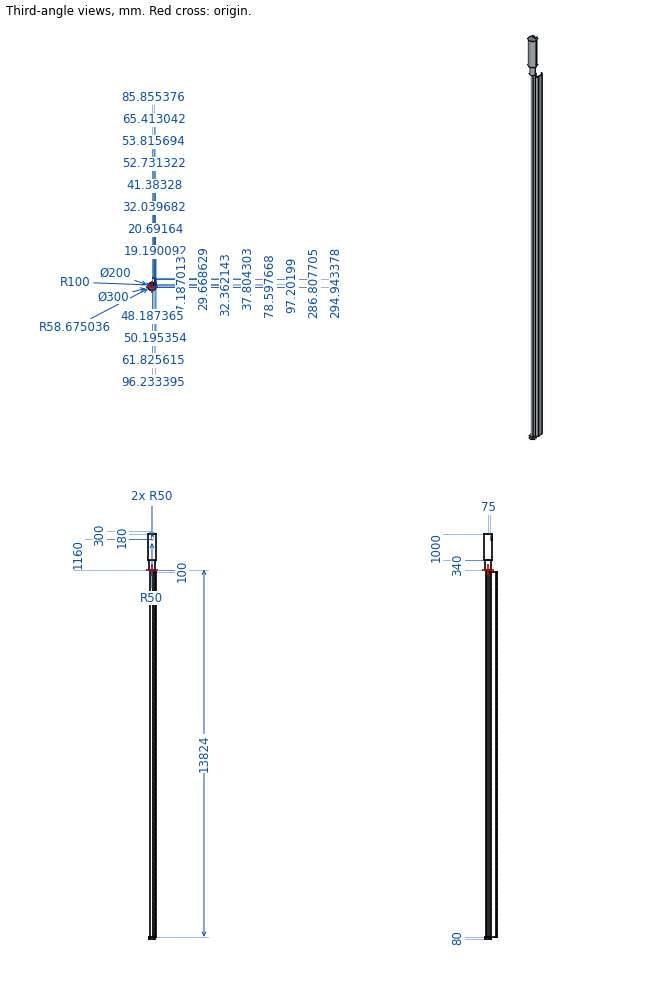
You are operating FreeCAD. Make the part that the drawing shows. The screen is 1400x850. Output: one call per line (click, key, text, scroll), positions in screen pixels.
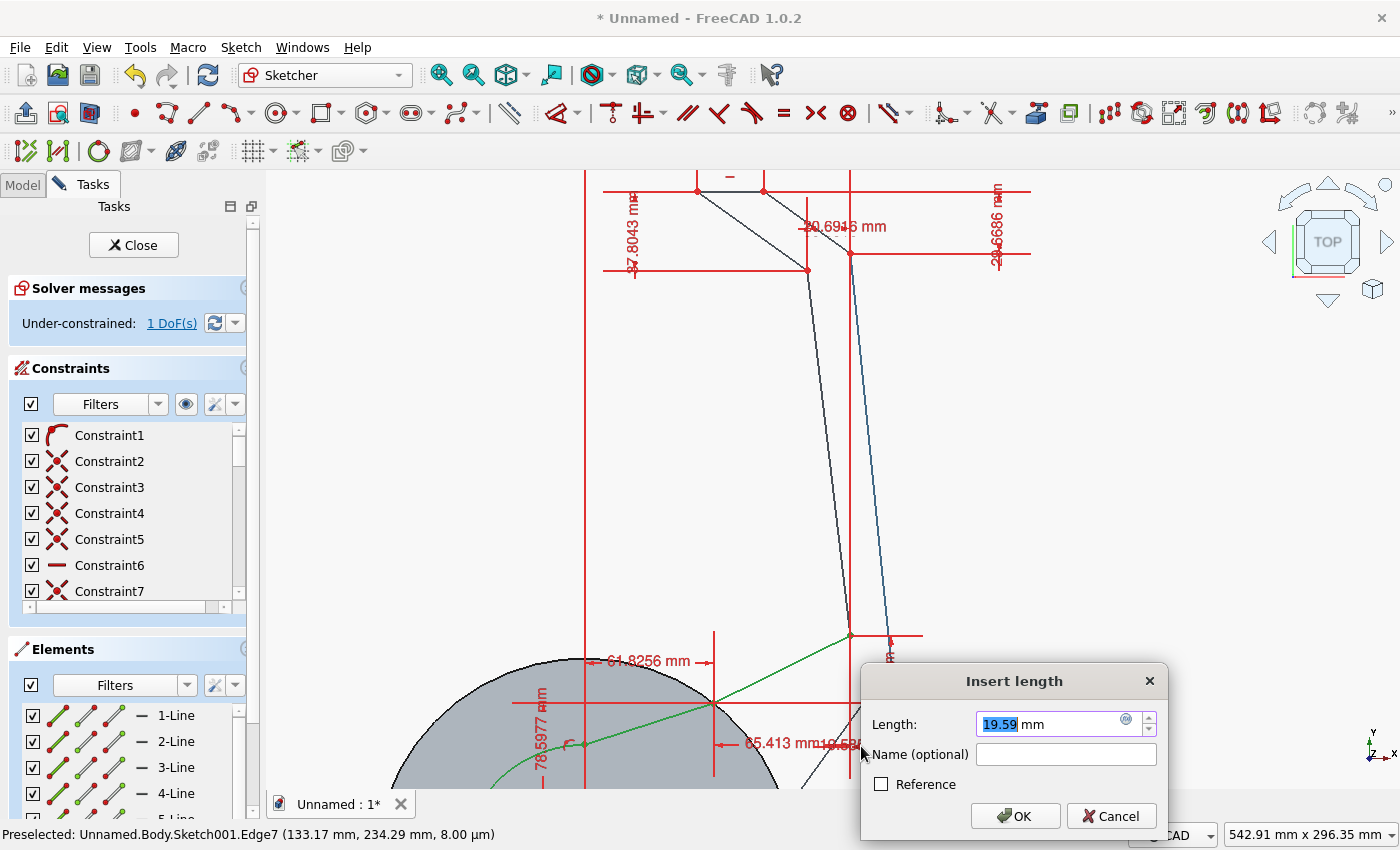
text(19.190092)
key(Return)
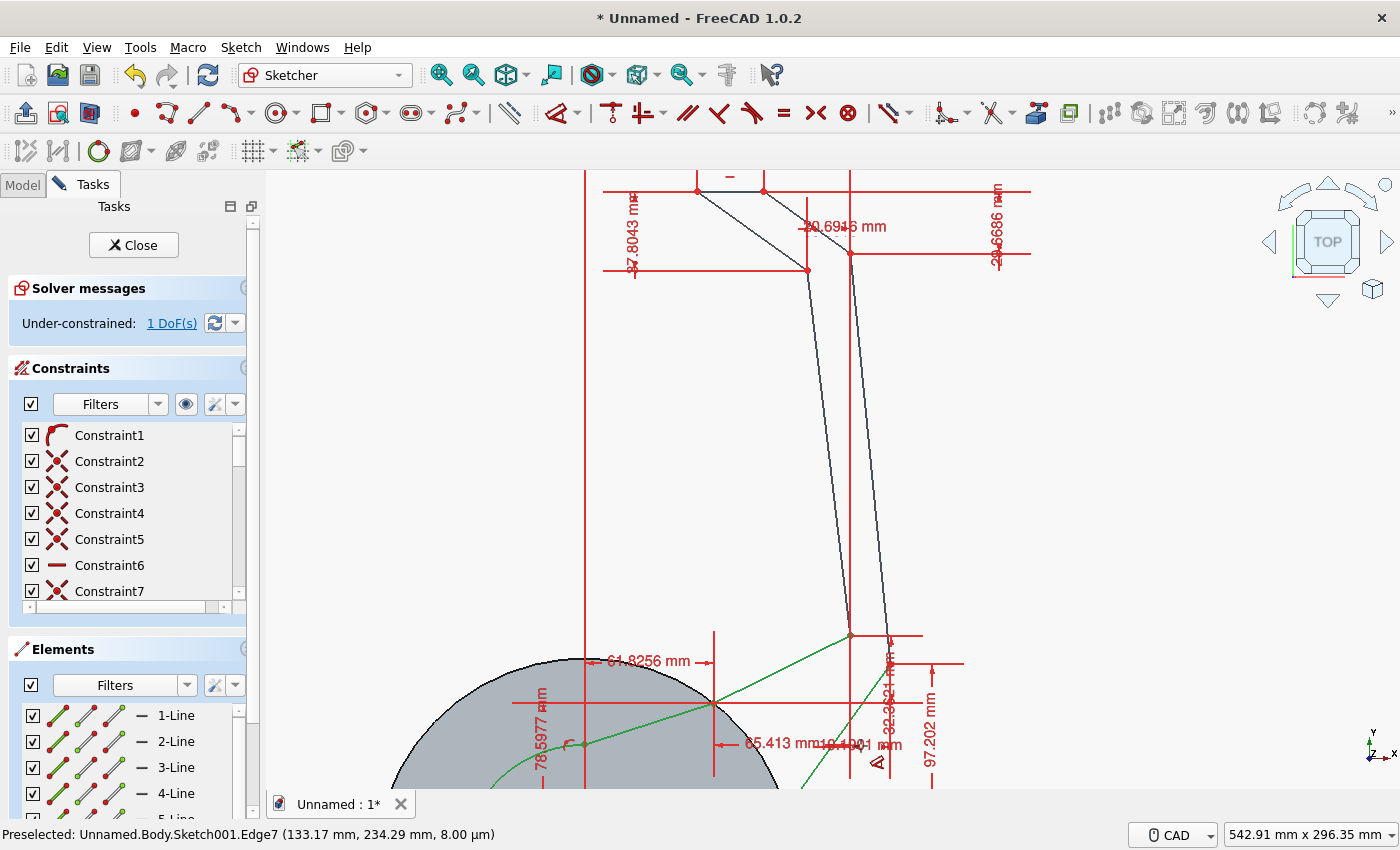
click(807, 271)
click(841, 403)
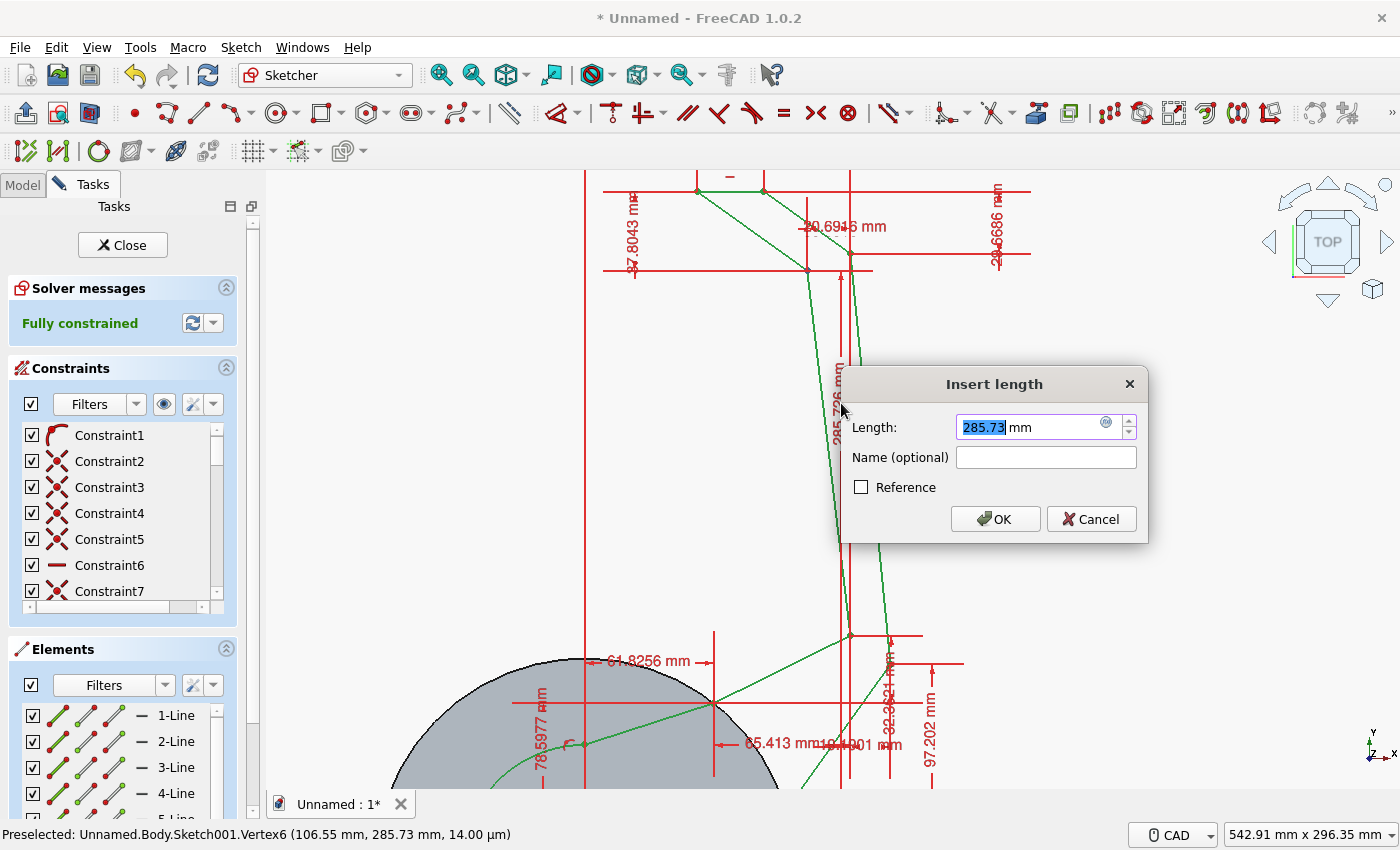
text(286.807705)
key(Return)
key(Escape)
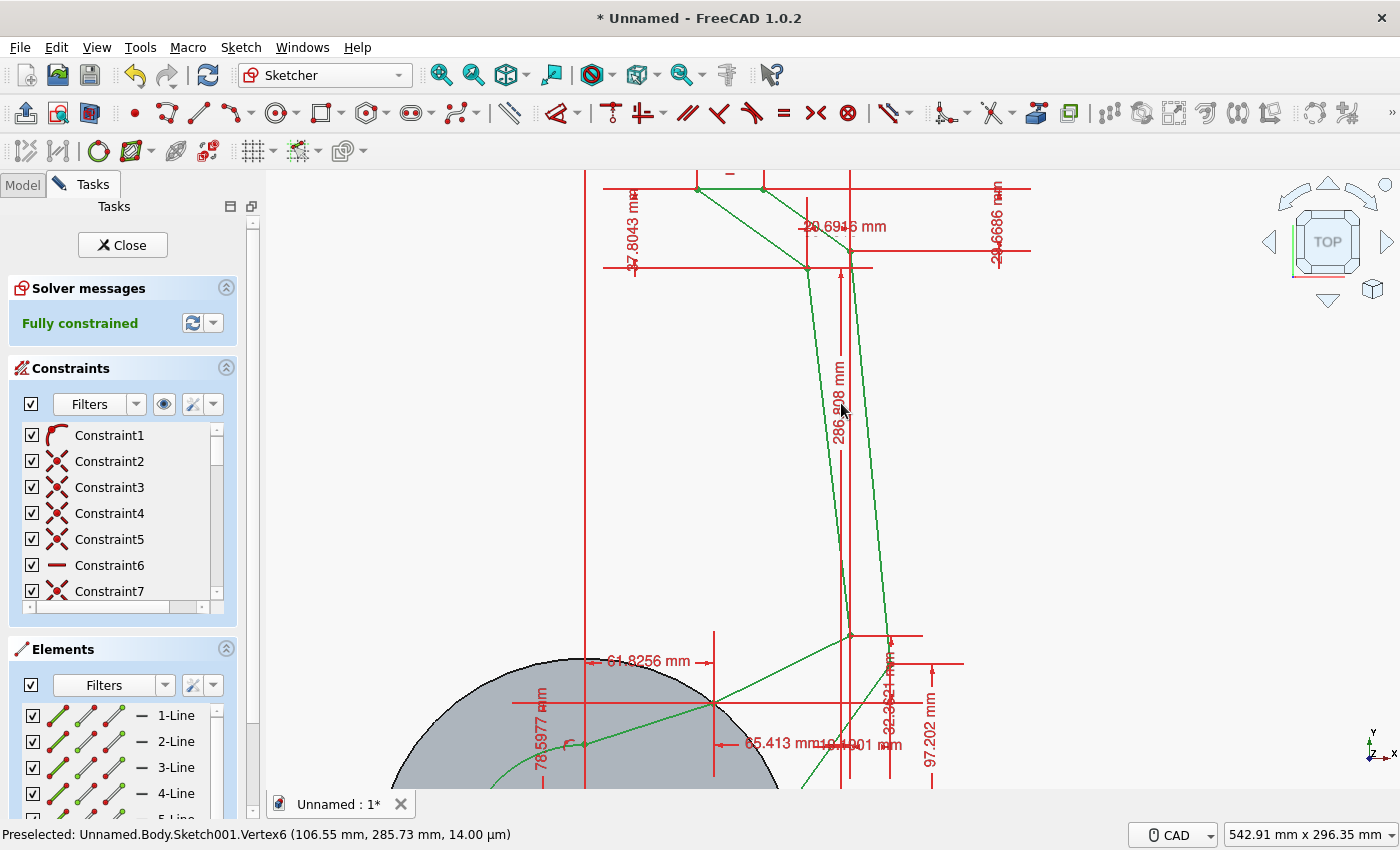
click(123, 245)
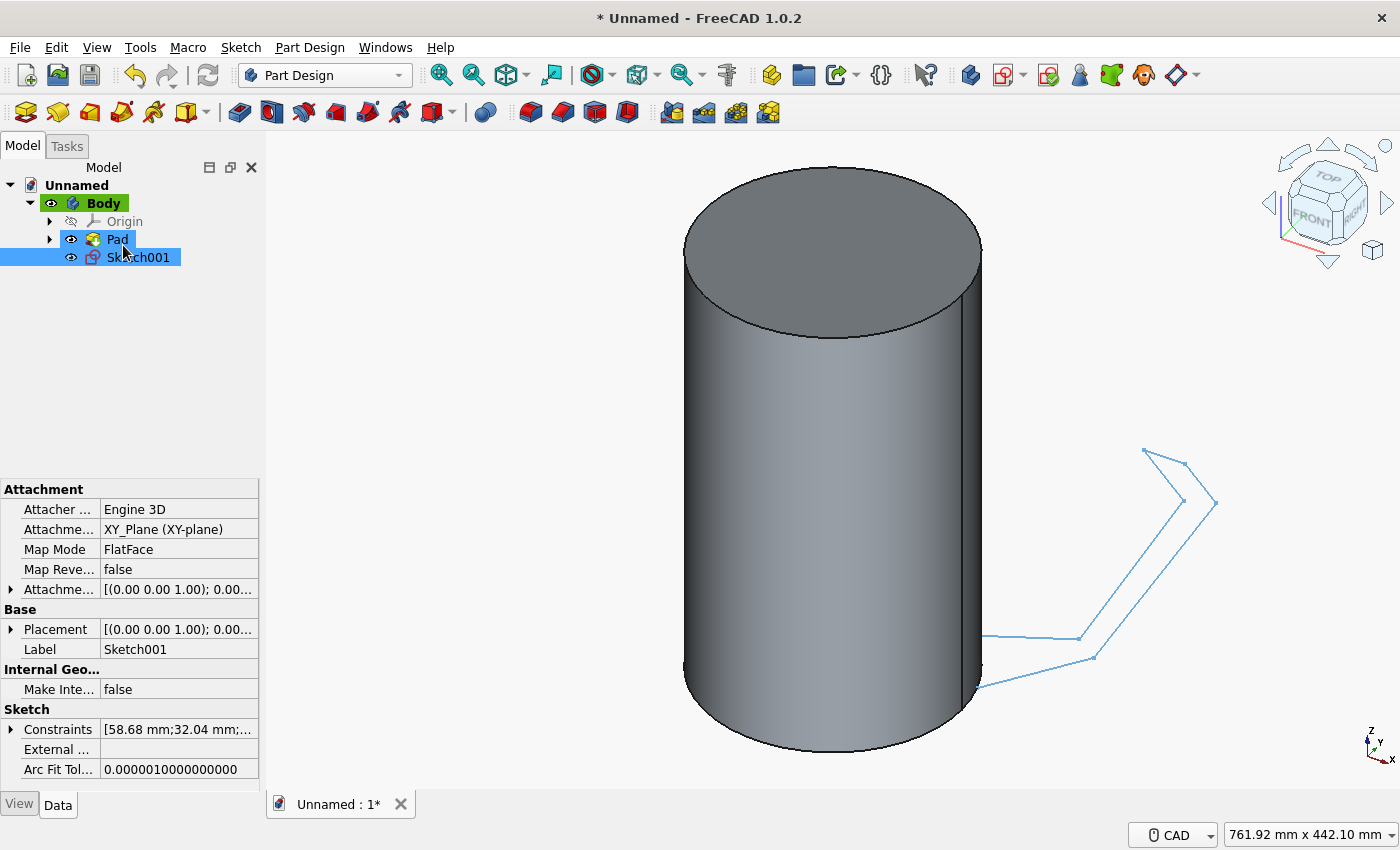
click(26, 112)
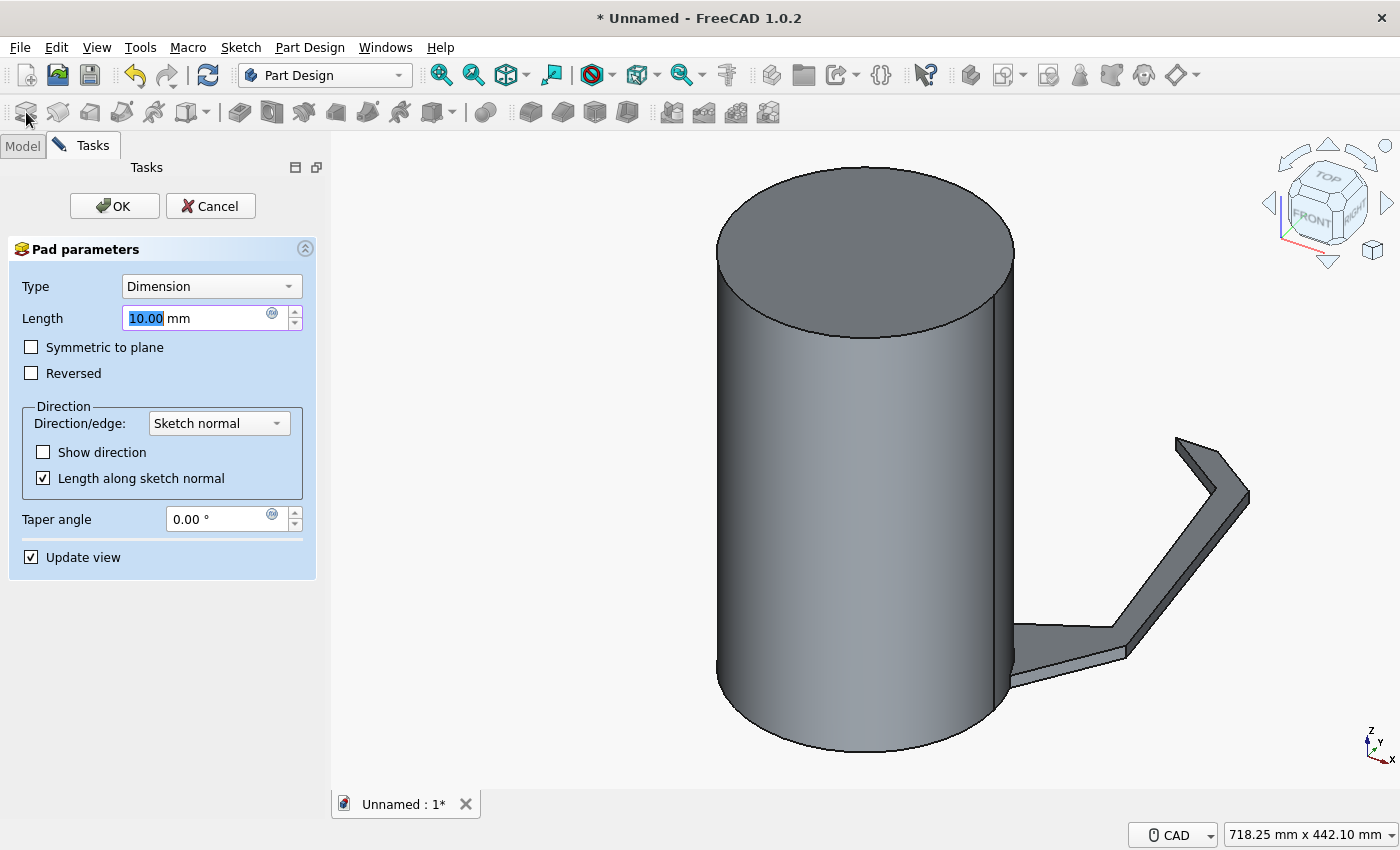
text(13824)
key(Tab)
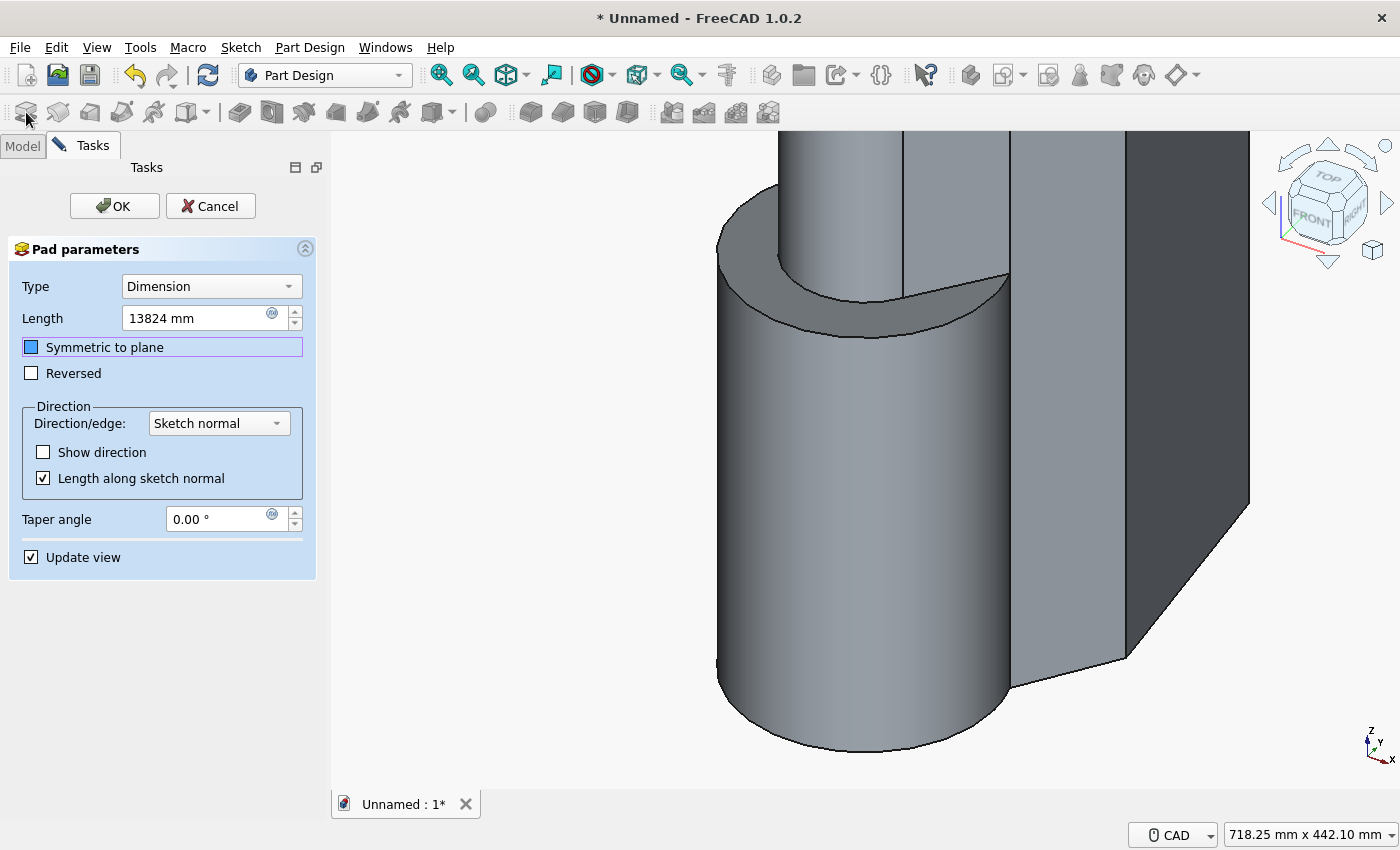
click(30, 373)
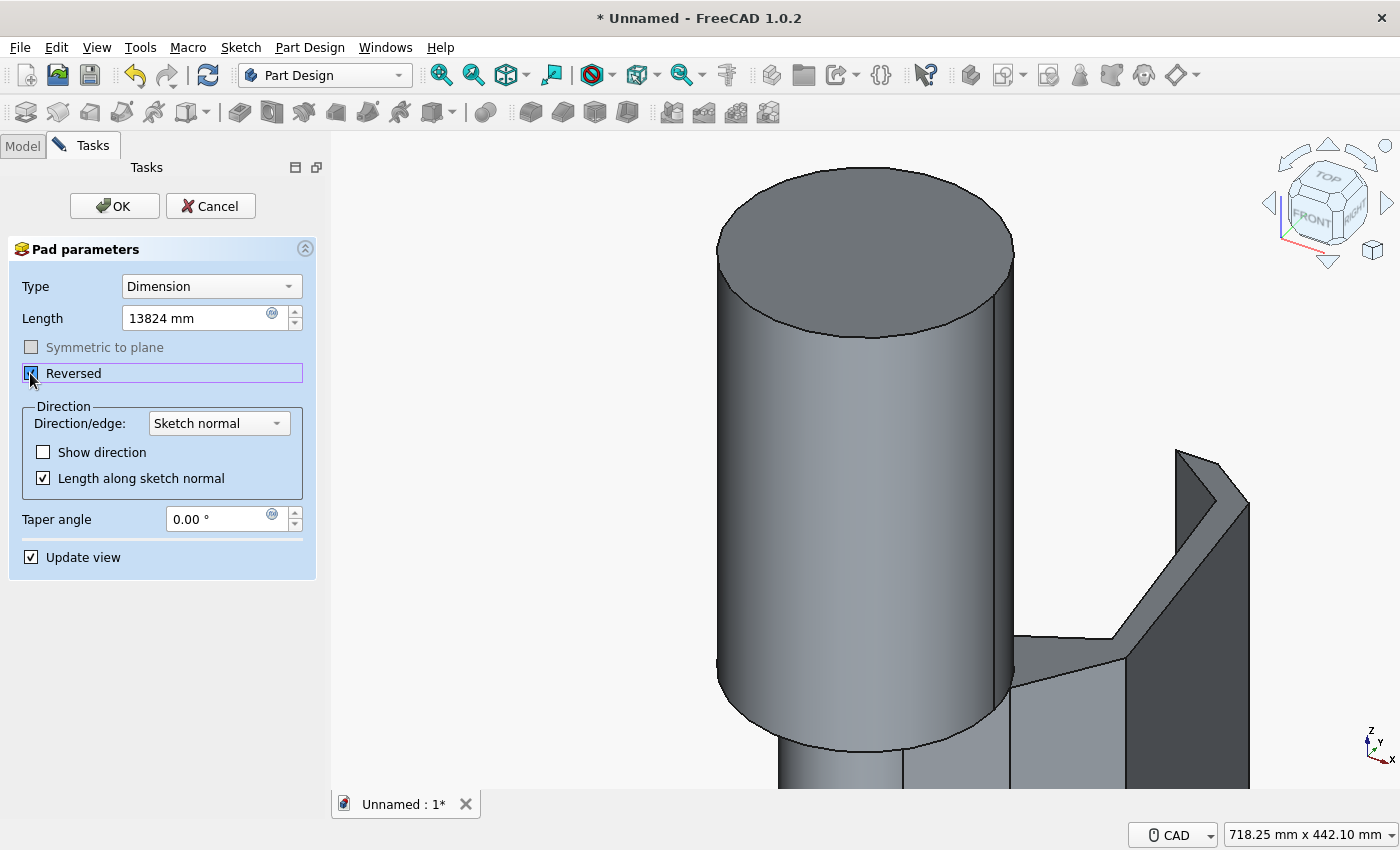
click(115, 206)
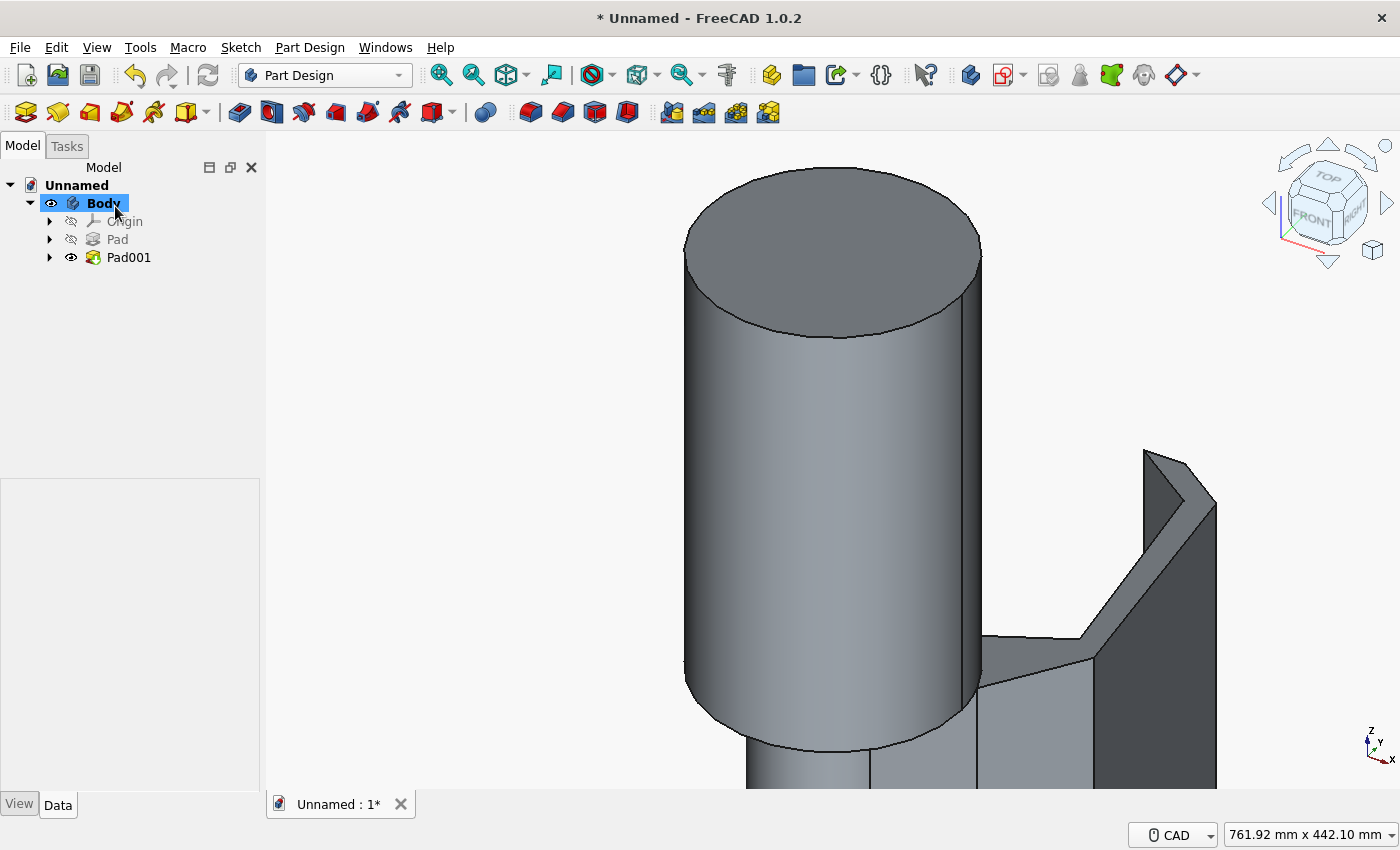
key(v)
key(f)